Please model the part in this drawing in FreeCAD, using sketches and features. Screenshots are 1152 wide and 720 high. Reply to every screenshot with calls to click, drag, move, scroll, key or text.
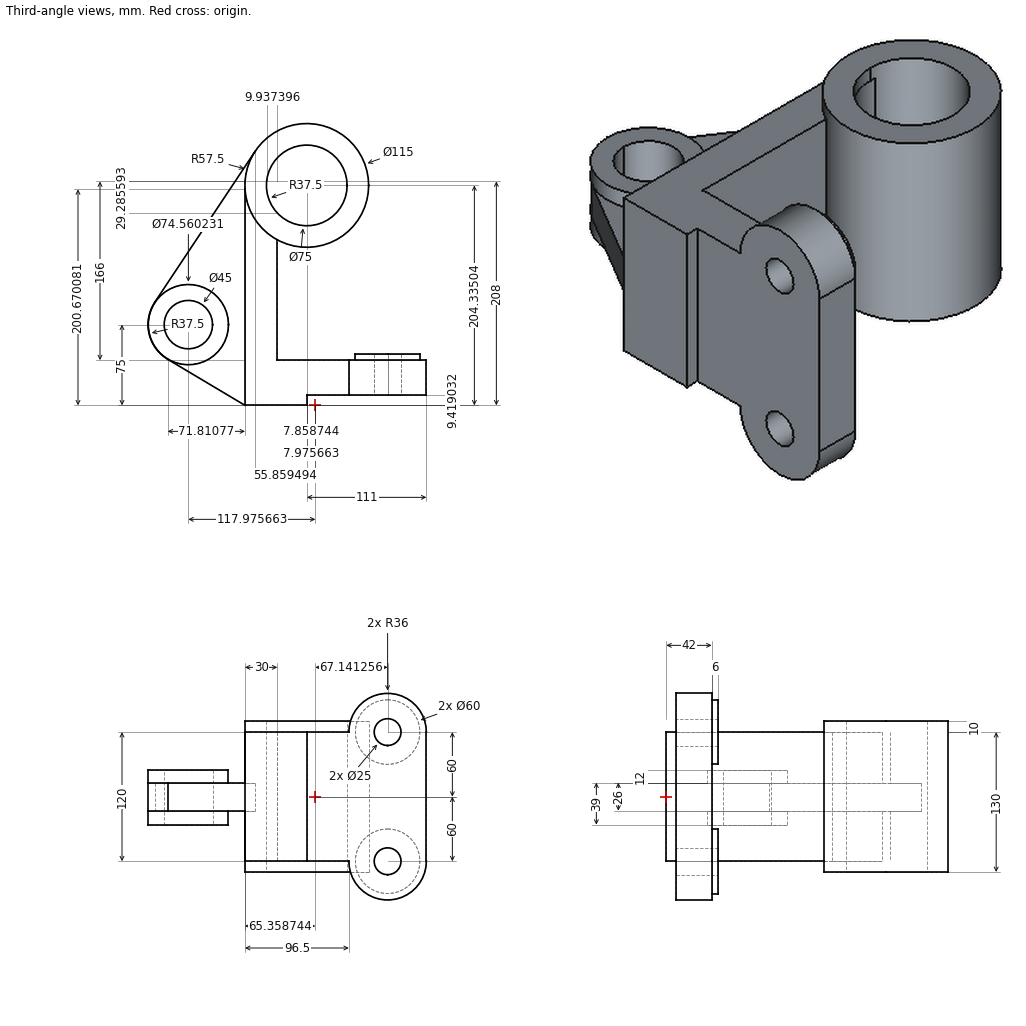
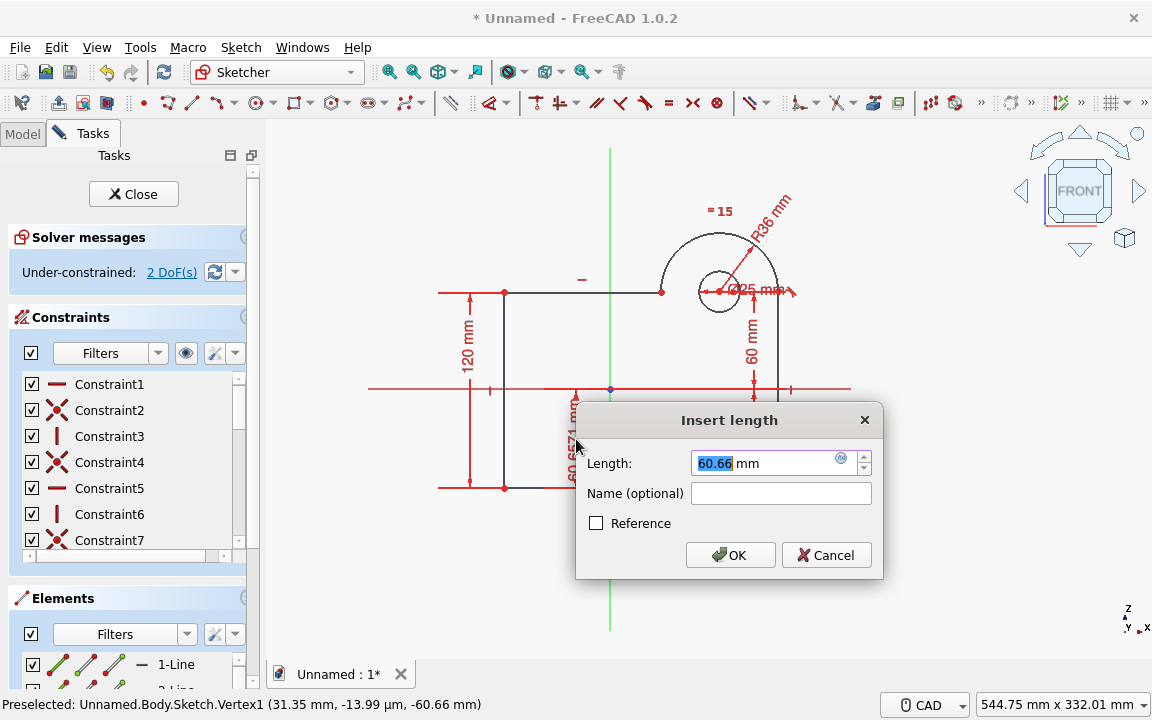
text(60)
key(Return)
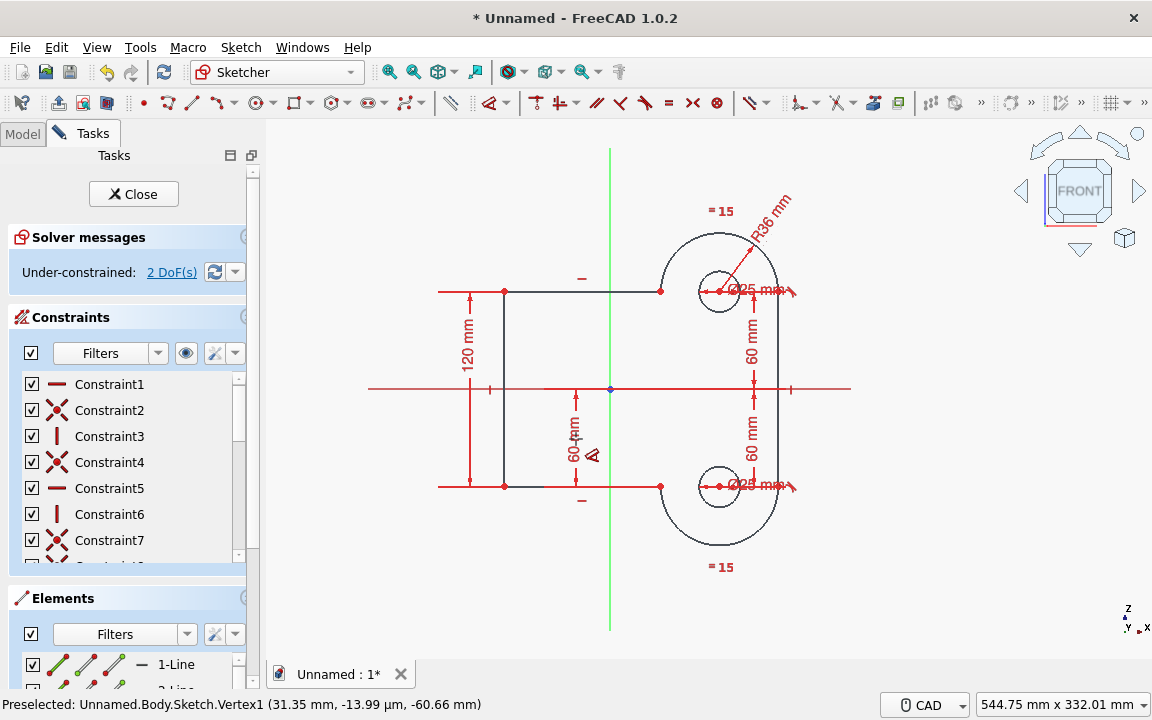
click(614, 487)
click(582, 521)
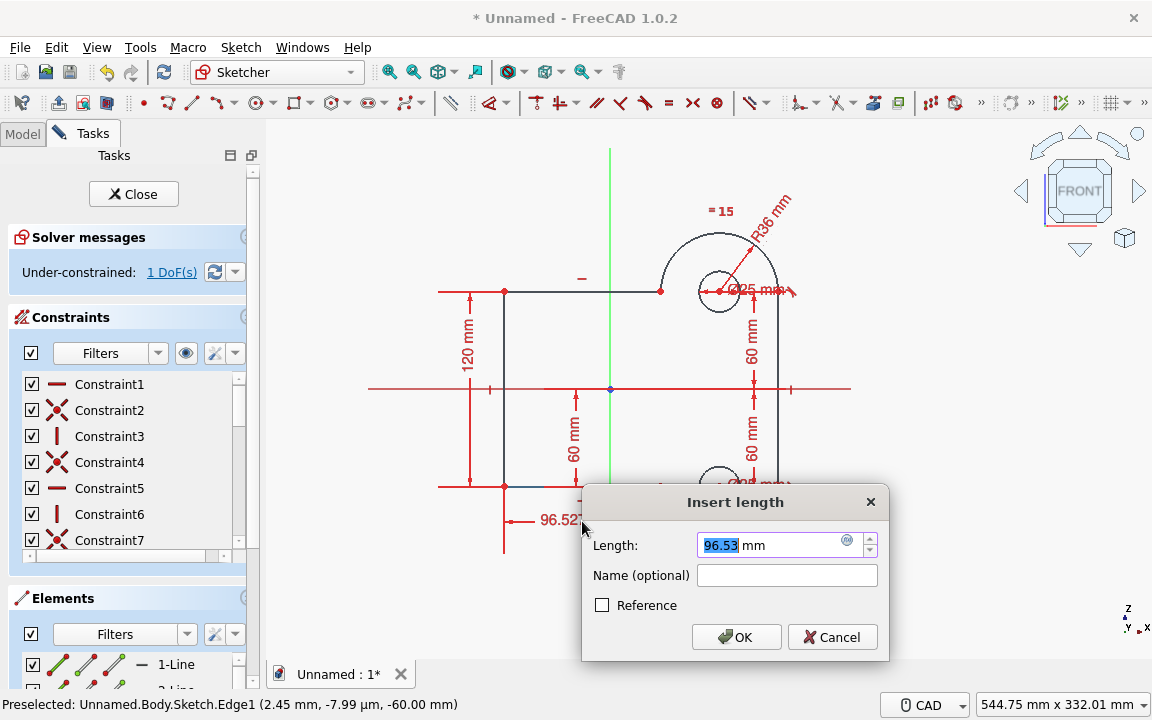
text(96.5)
key(Return)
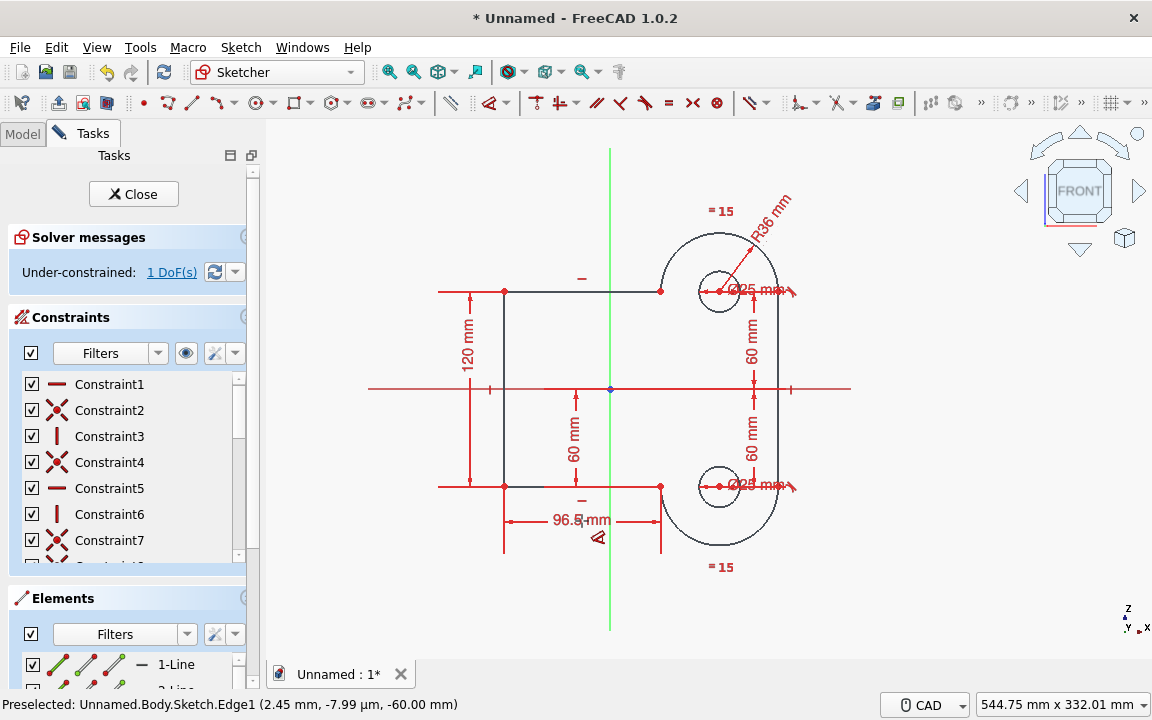
click(720, 292)
click(640, 258)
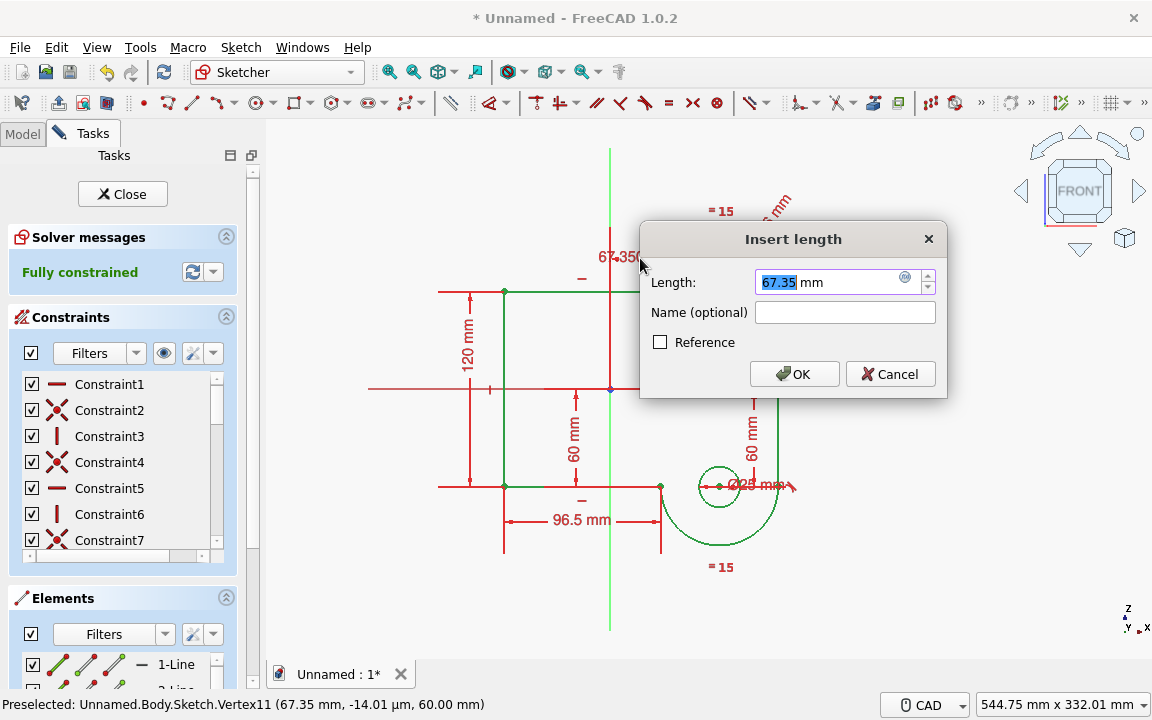
text(67.141256)
key(Return)
key(Escape)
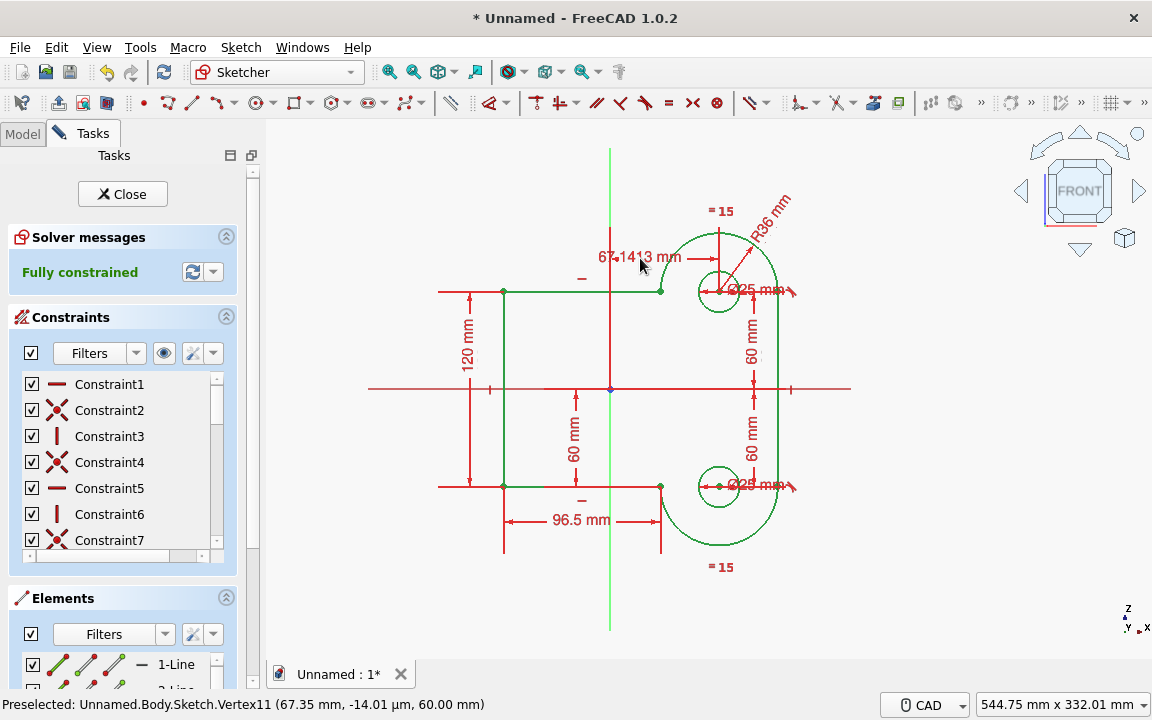
click(123, 194)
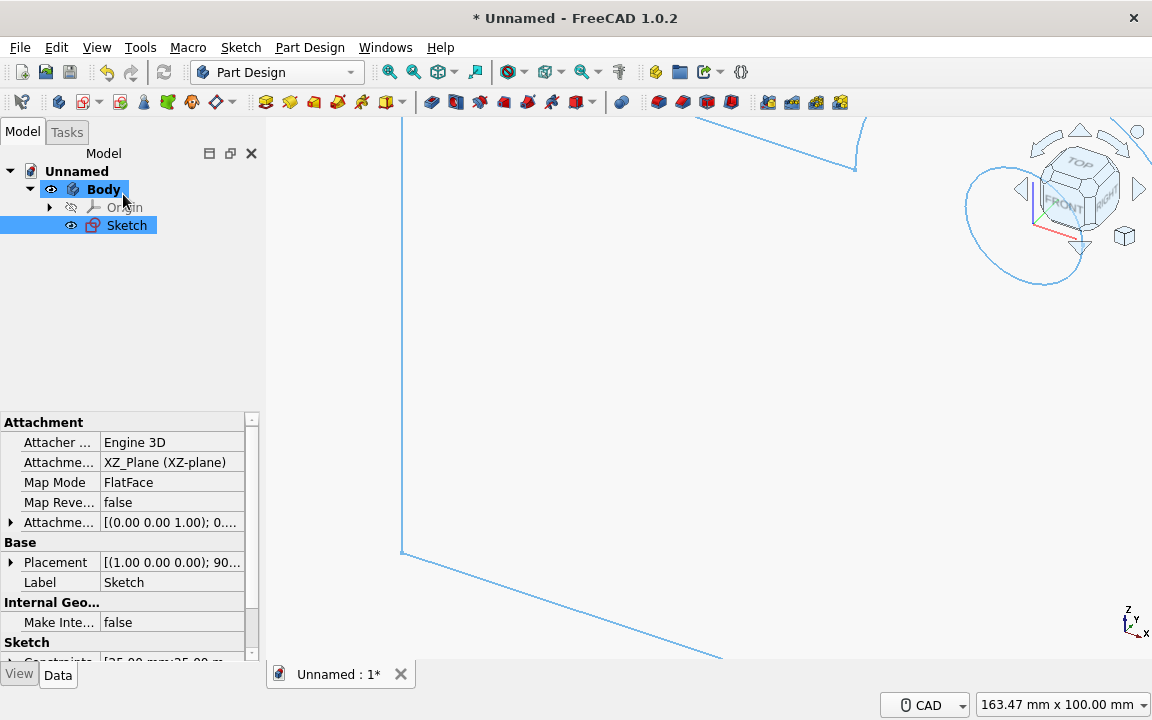
click(266, 102)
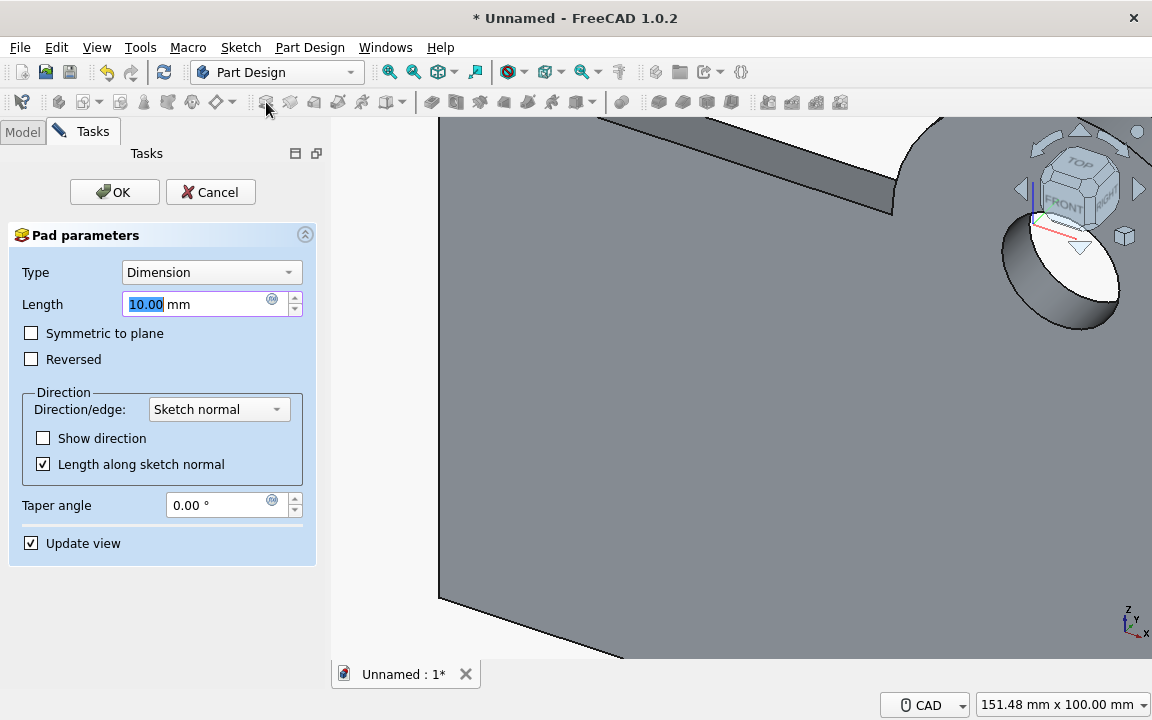
text(42)
key(Tab)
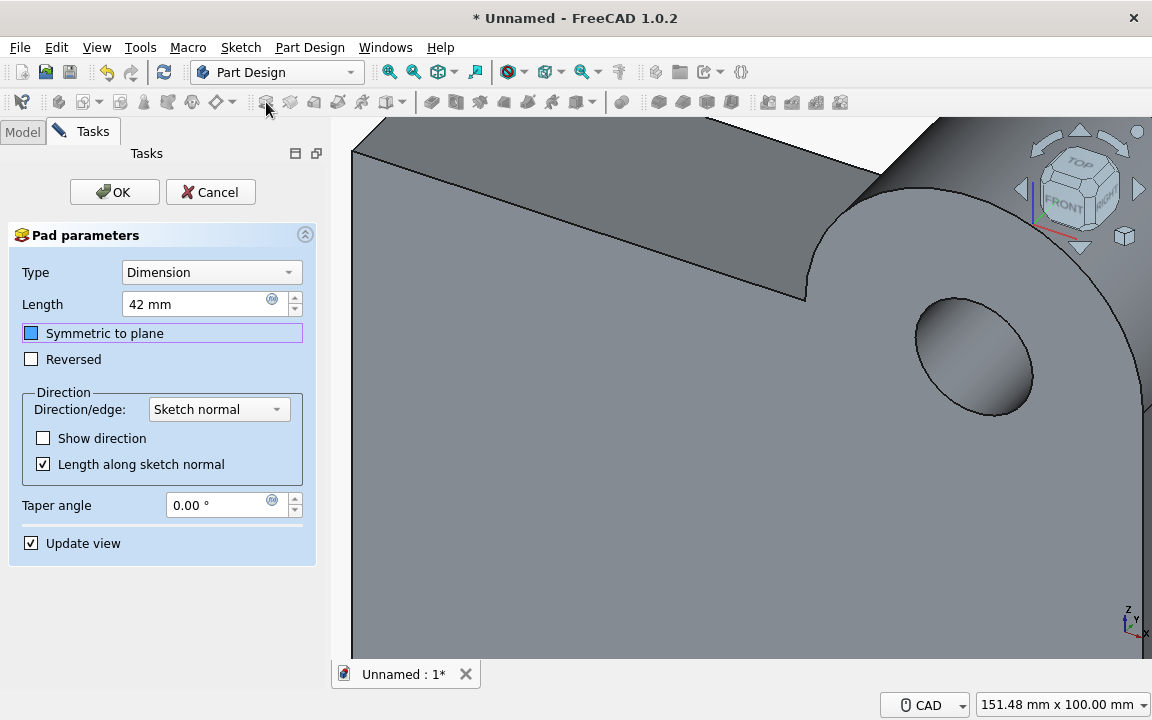
click(30, 359)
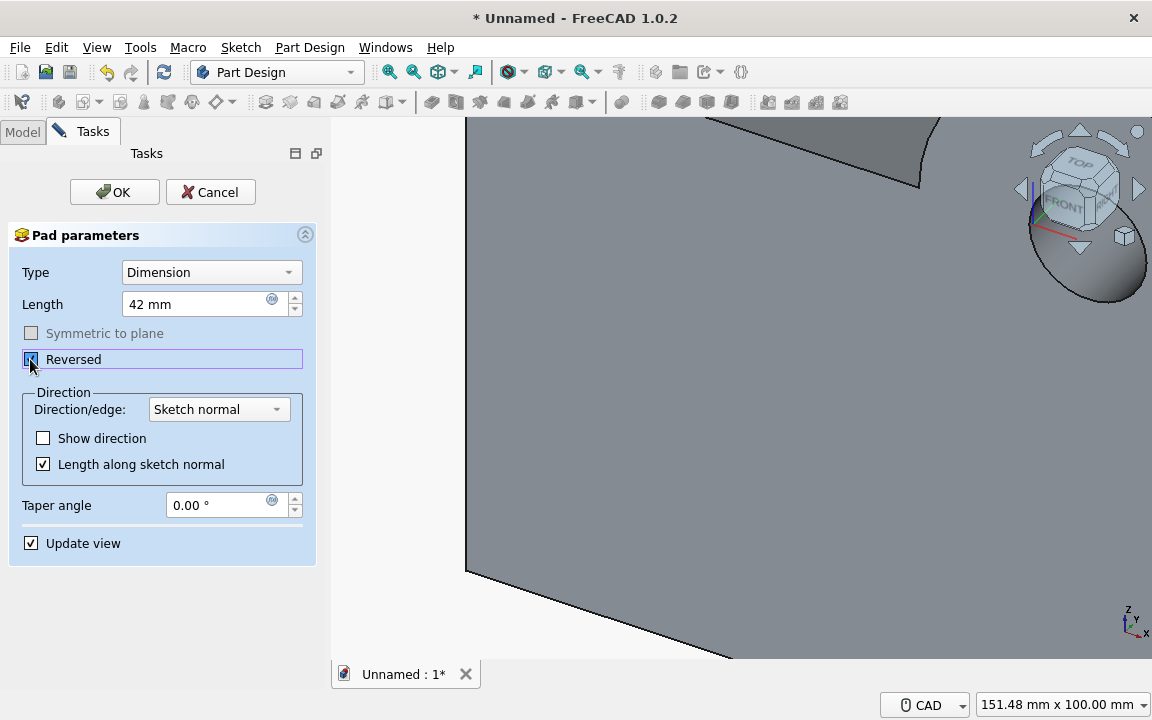
click(115, 192)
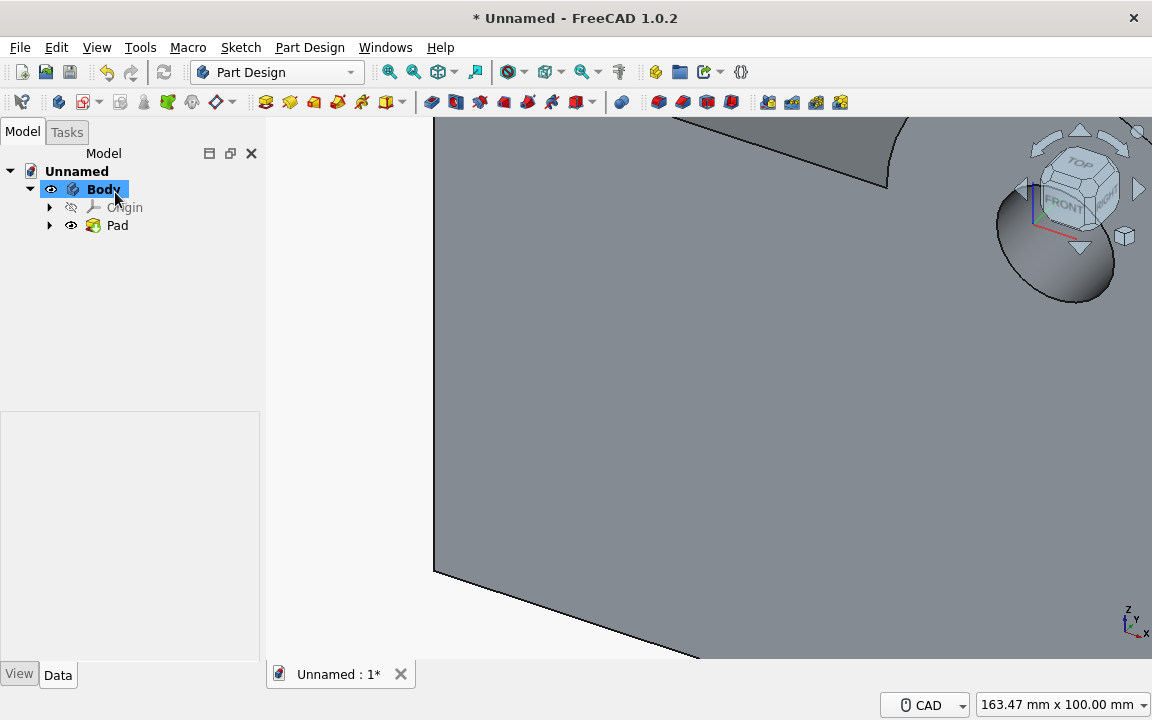
click(390, 72)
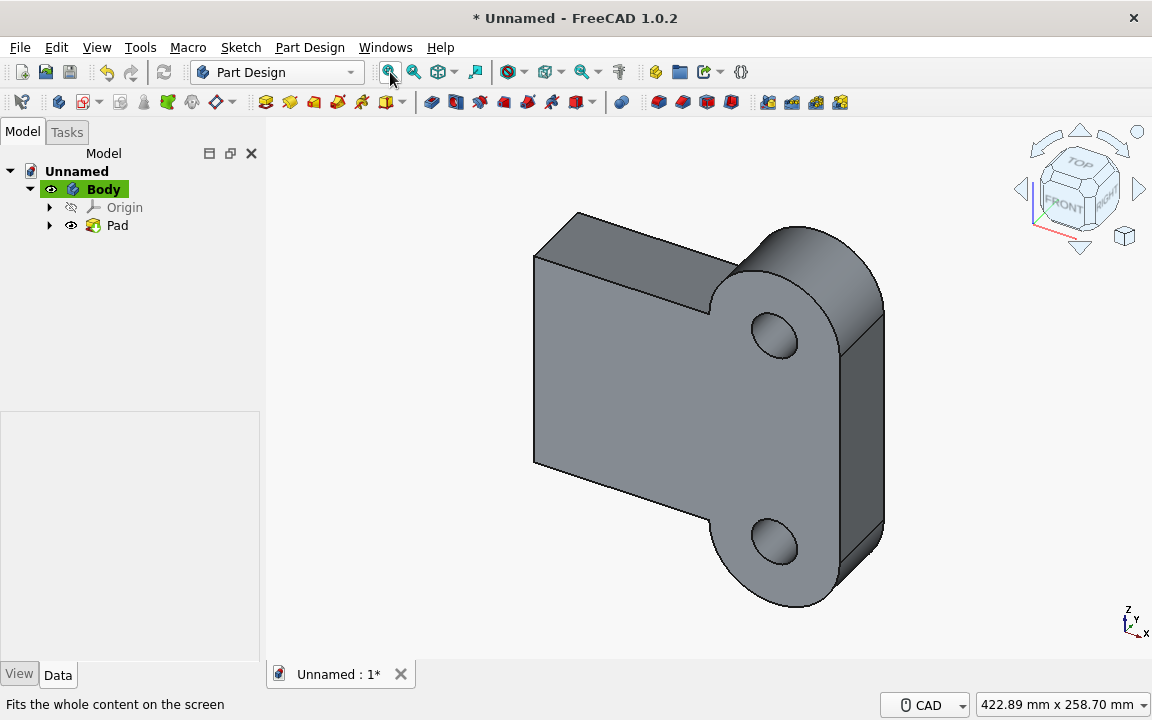
key(4)